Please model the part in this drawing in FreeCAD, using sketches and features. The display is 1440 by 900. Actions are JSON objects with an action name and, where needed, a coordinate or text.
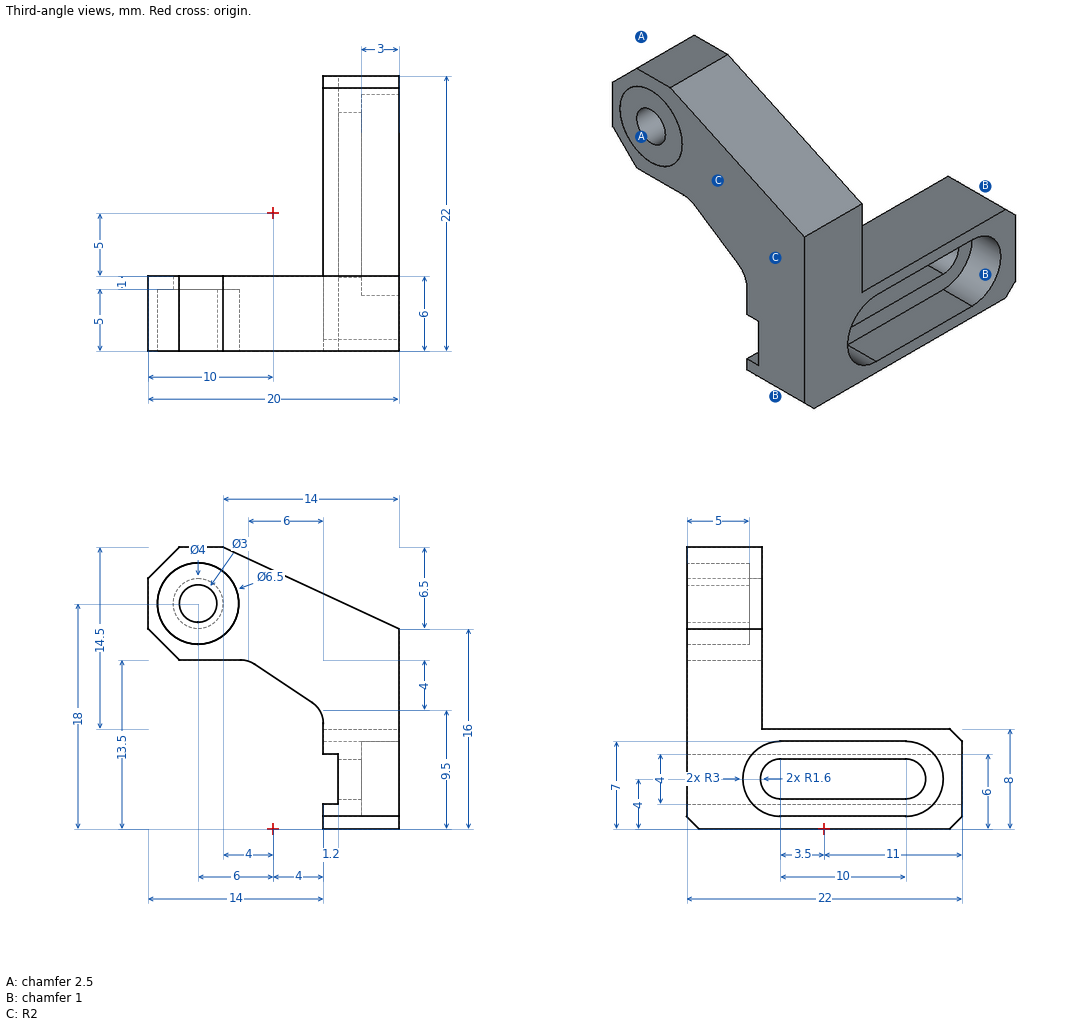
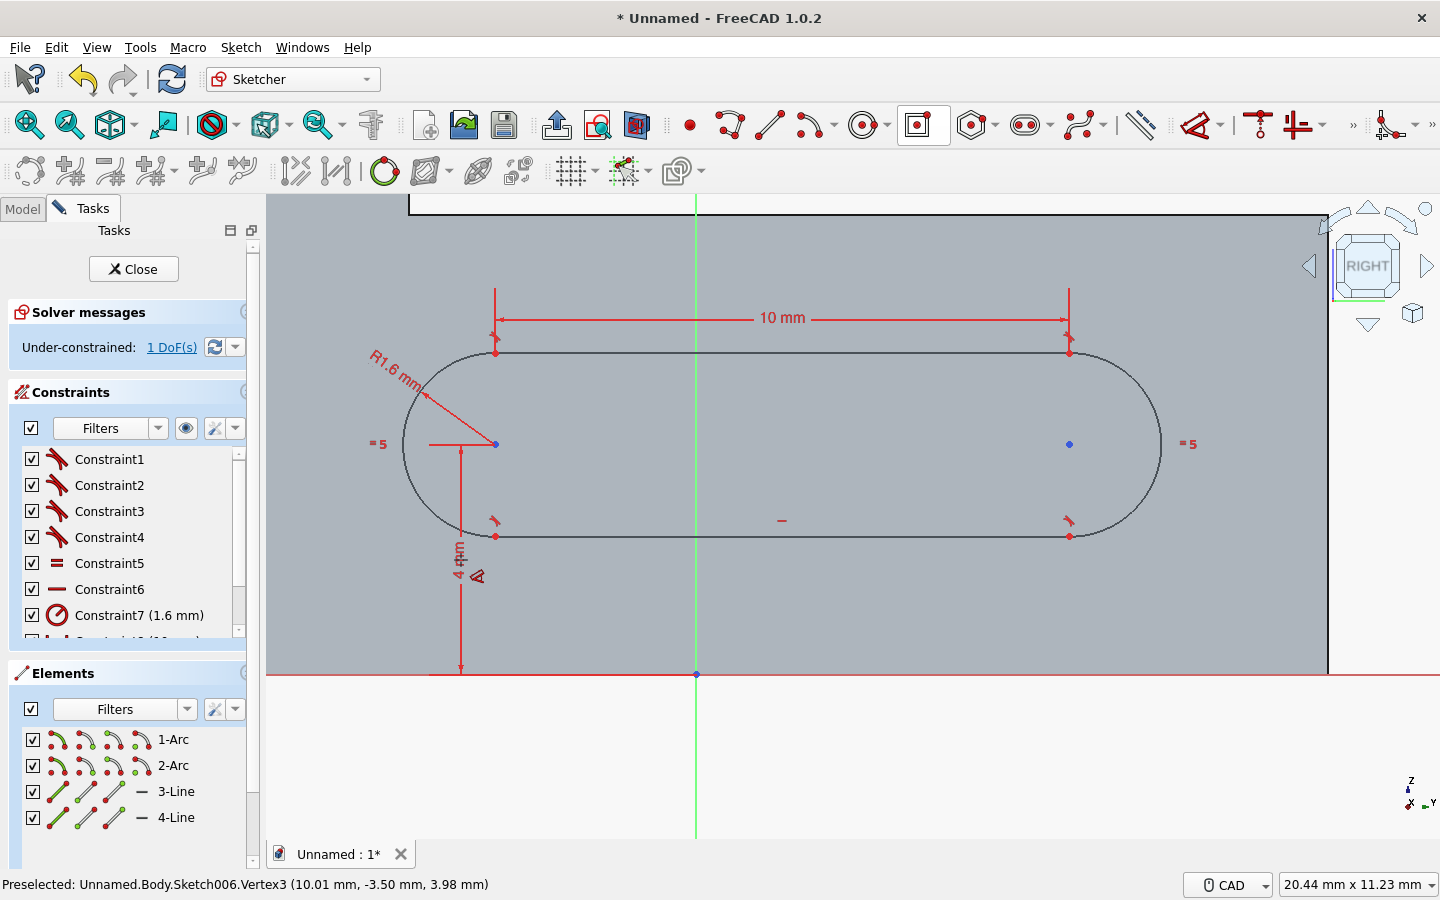
{"action": "left_click", "coordinate": [495, 353]}
{"action": "left_click", "coordinate": [596, 709]}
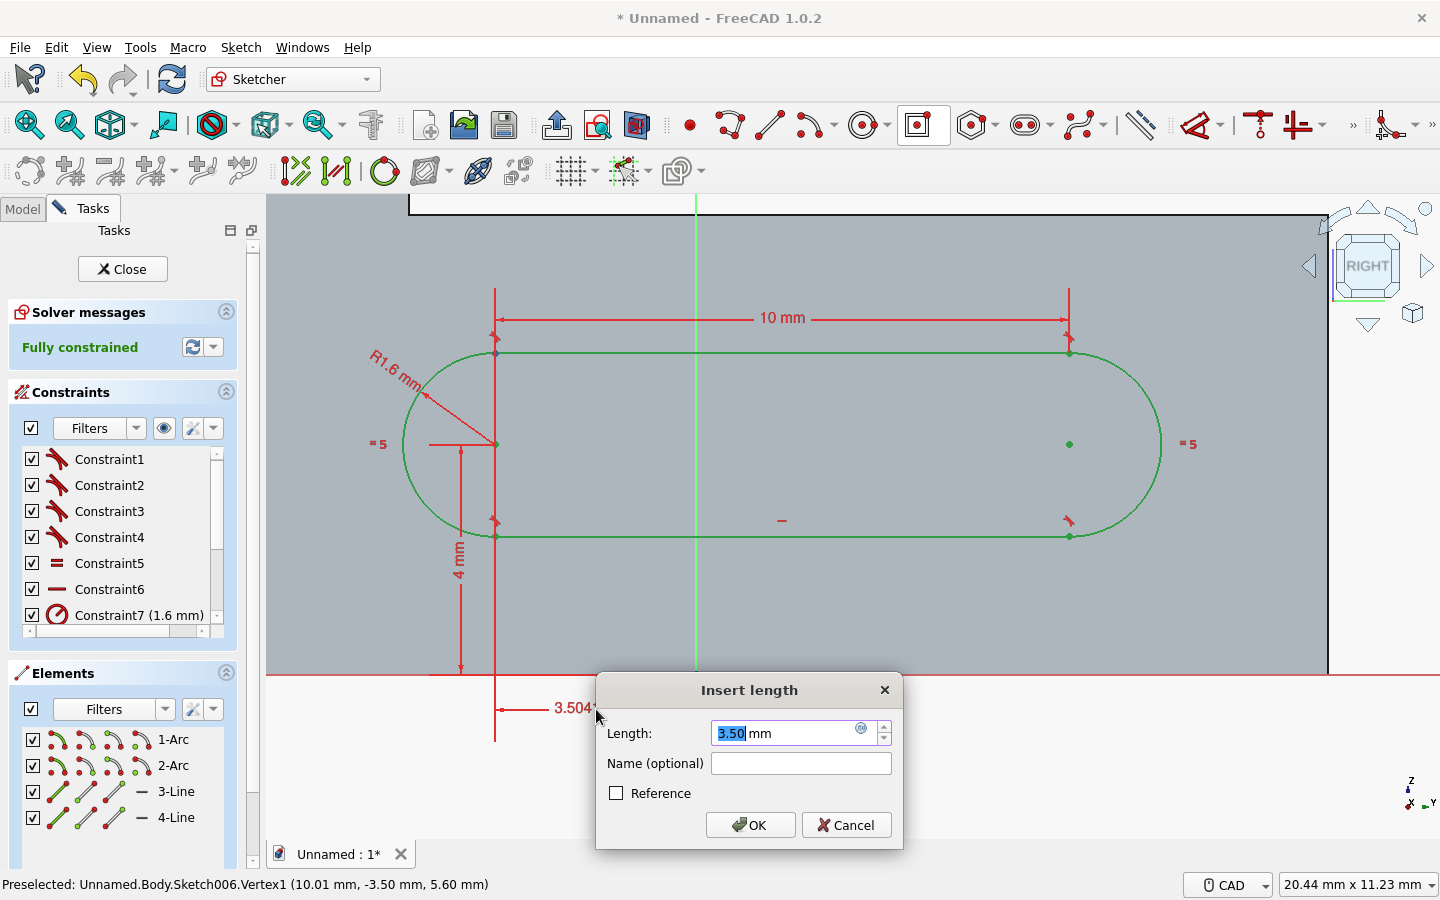
{"action": "type", "text": "3.5"}
{"action": "key", "text": "Return"}
{"action": "key", "text": "Escape"}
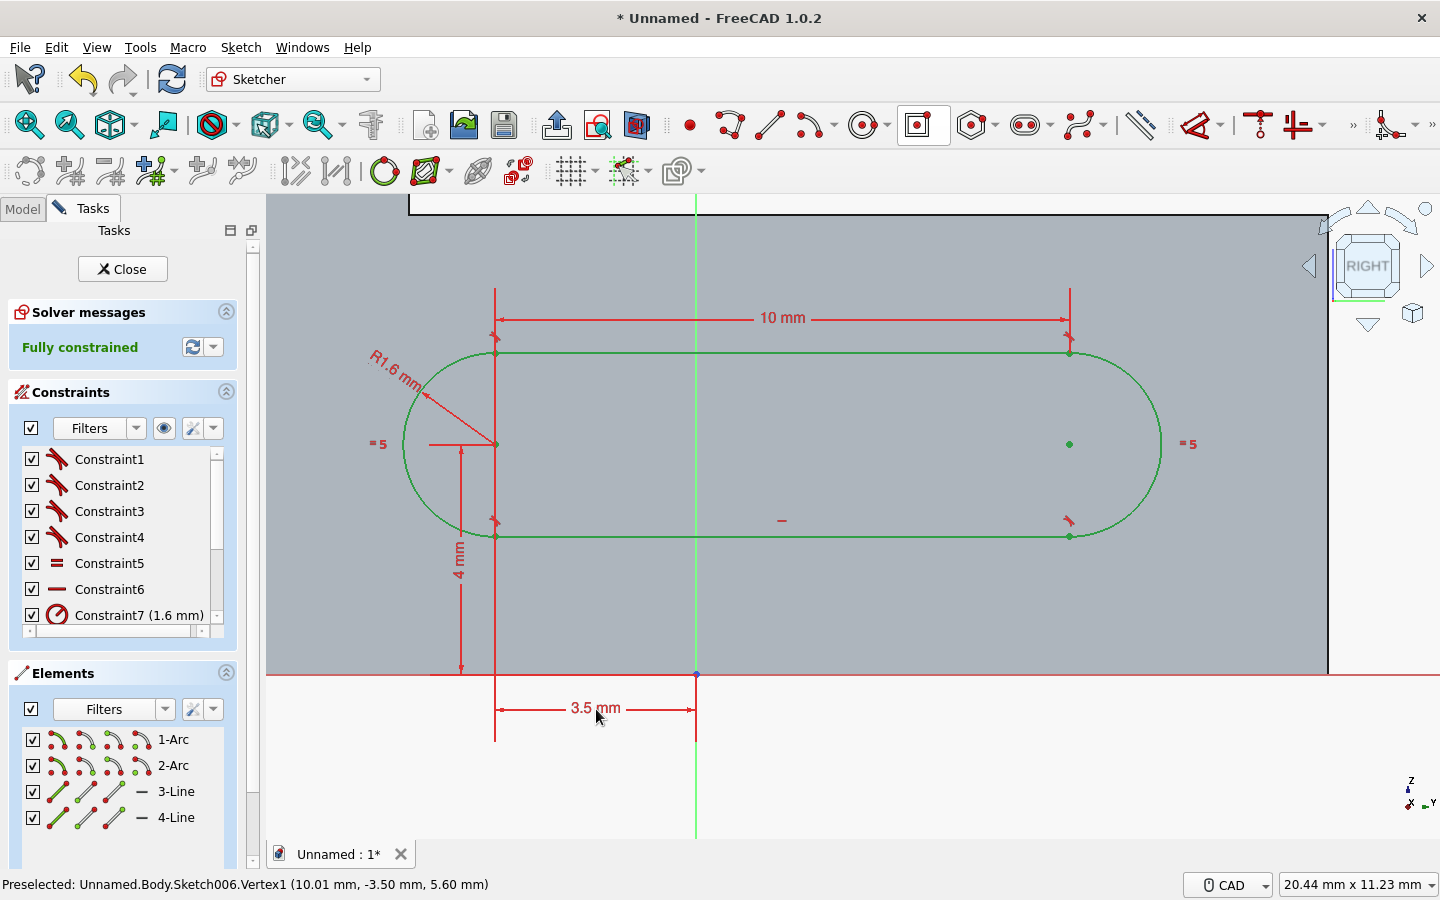
{"action": "left_click", "coordinate": [123, 269]}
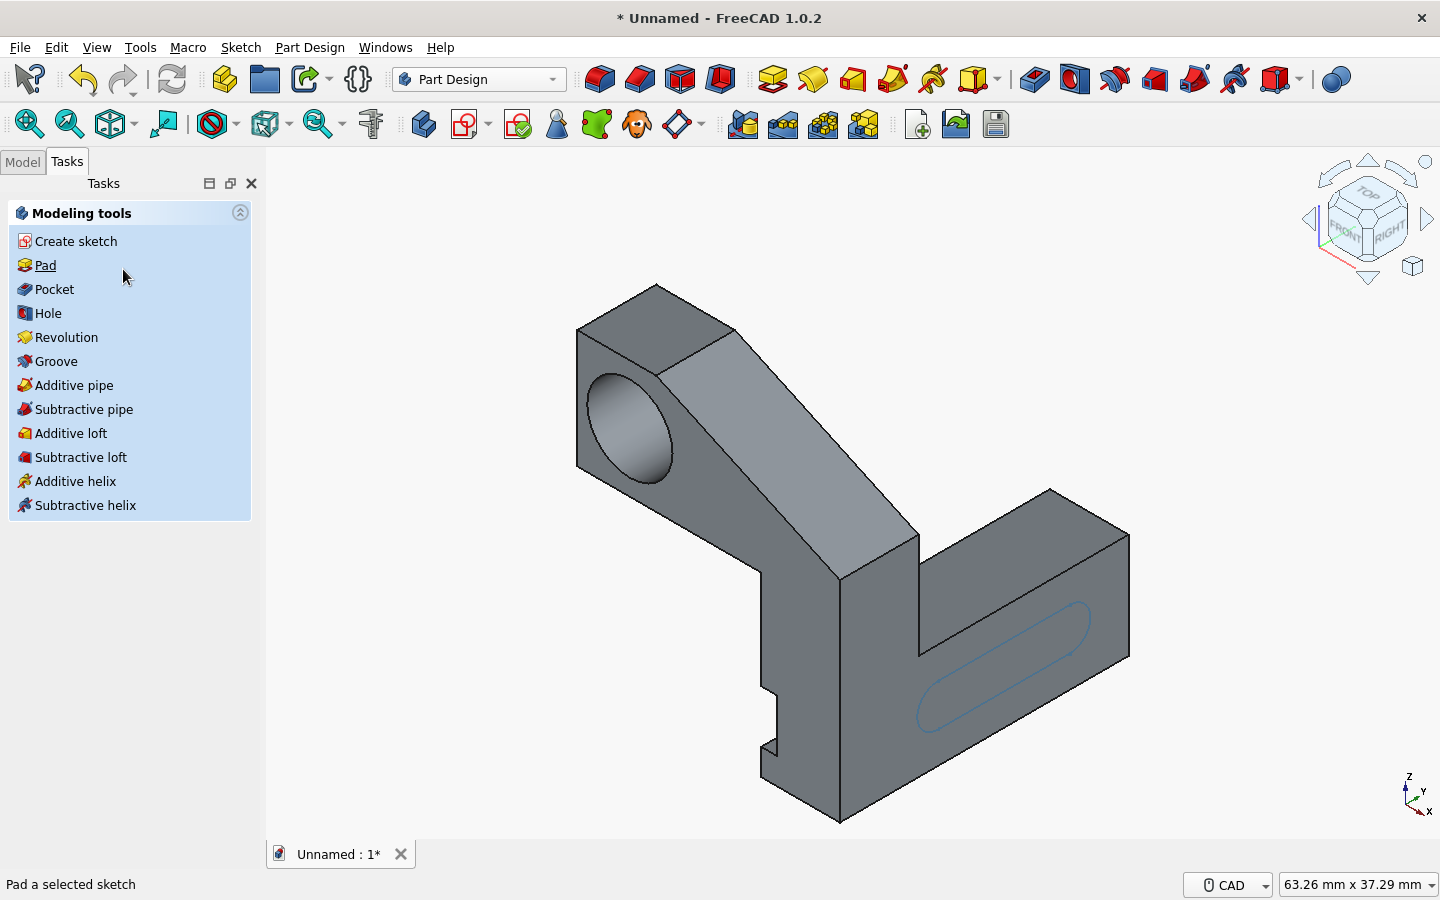
{"action": "left_click", "coordinate": [1036, 80]}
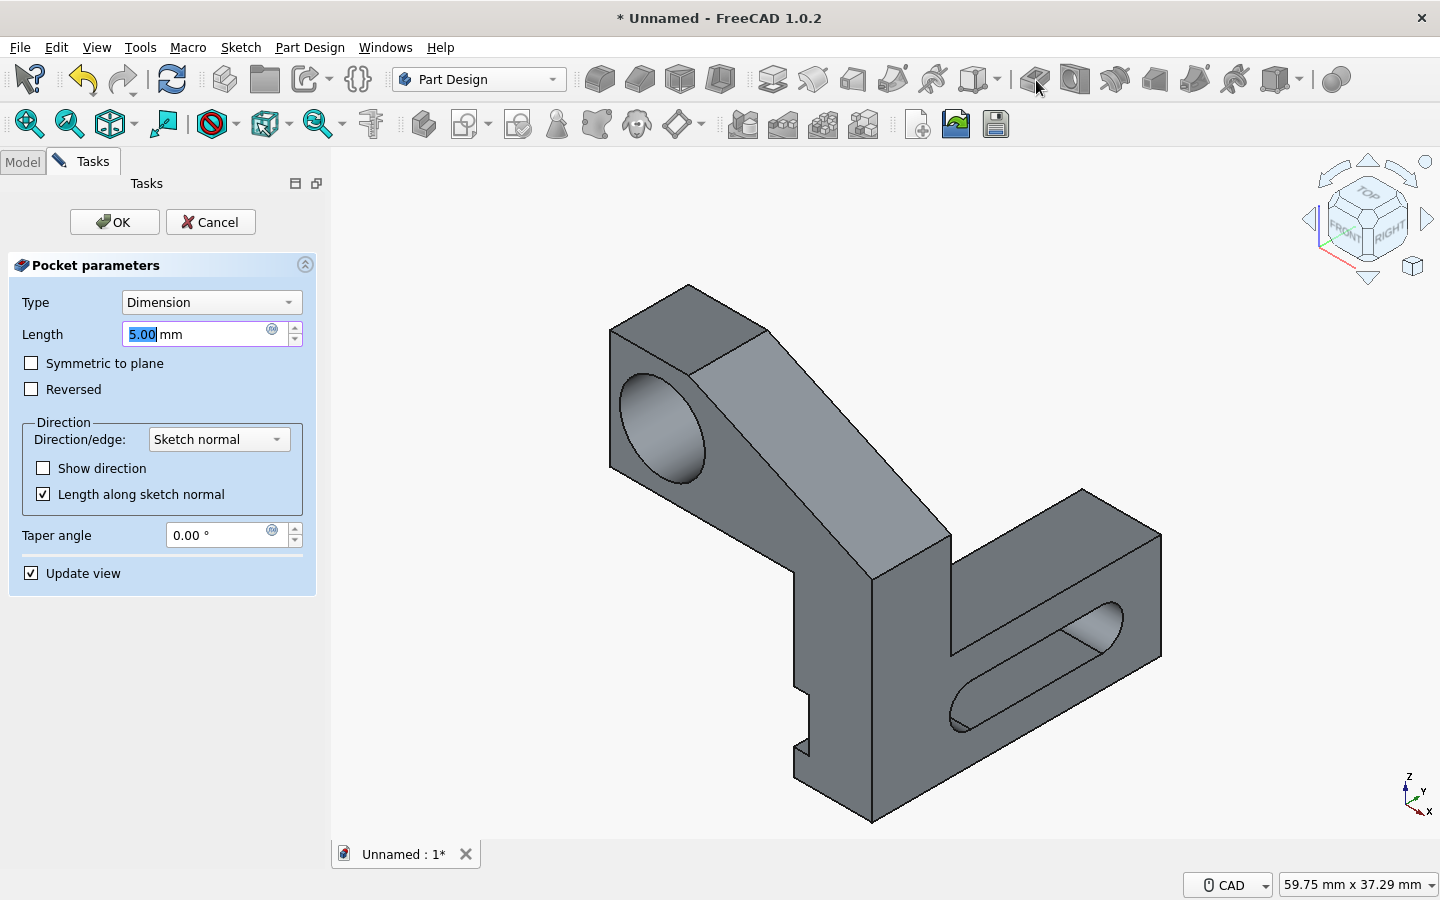
{"action": "left_click", "coordinate": [212, 302]}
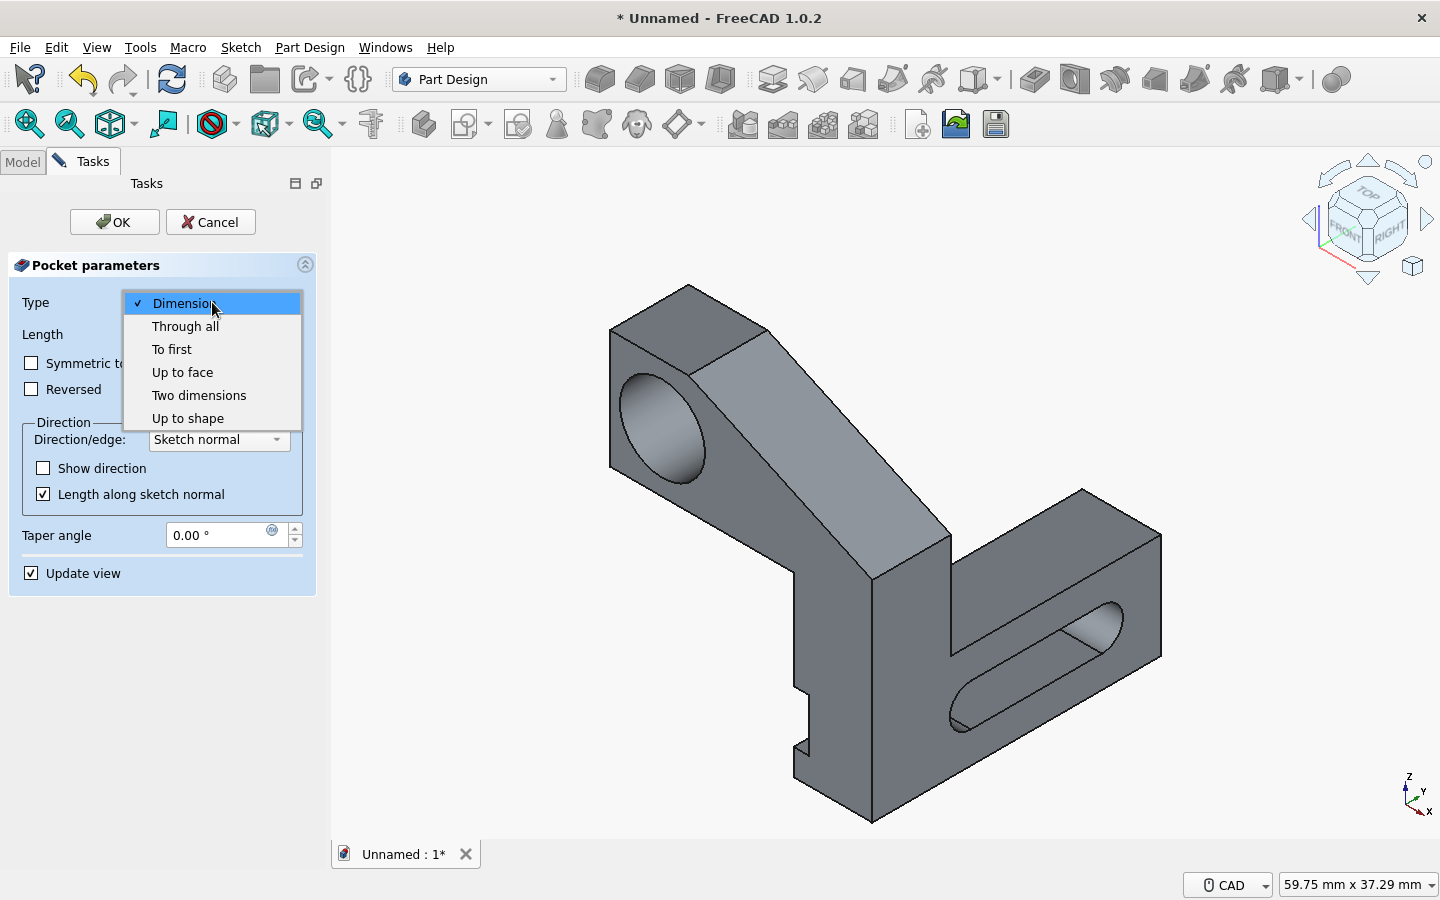
{"action": "left_click", "coordinate": [212, 326]}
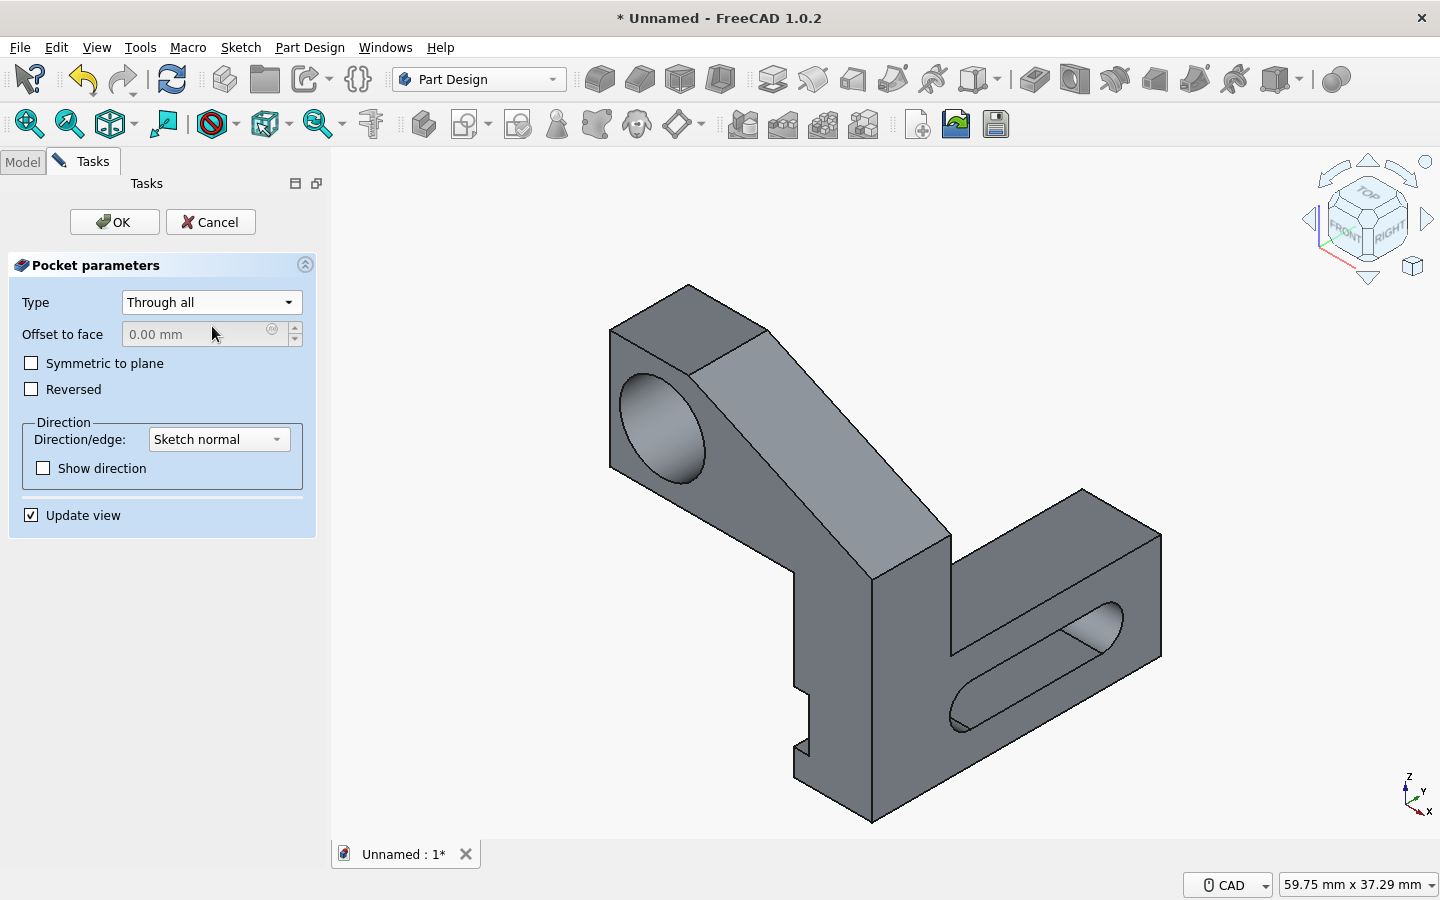
{"action": "left_click", "coordinate": [115, 222]}